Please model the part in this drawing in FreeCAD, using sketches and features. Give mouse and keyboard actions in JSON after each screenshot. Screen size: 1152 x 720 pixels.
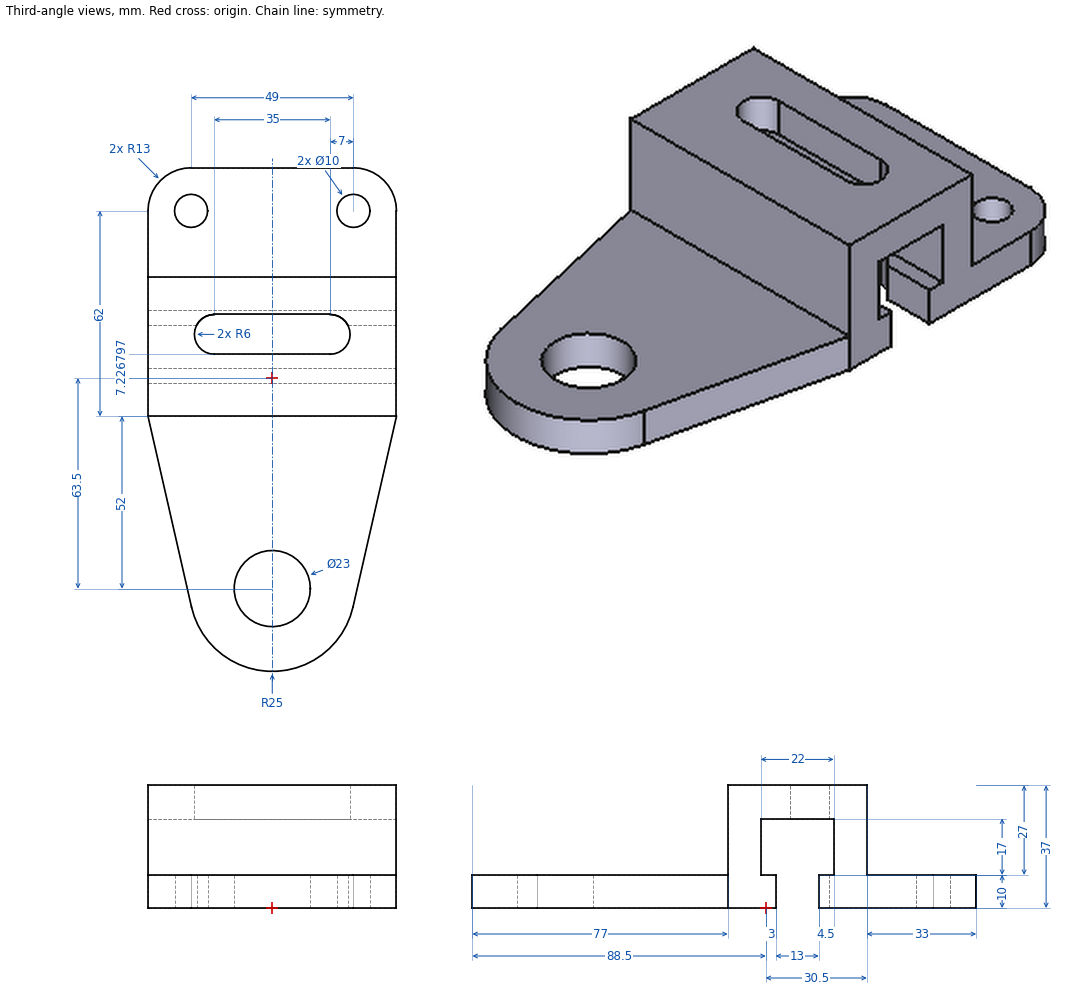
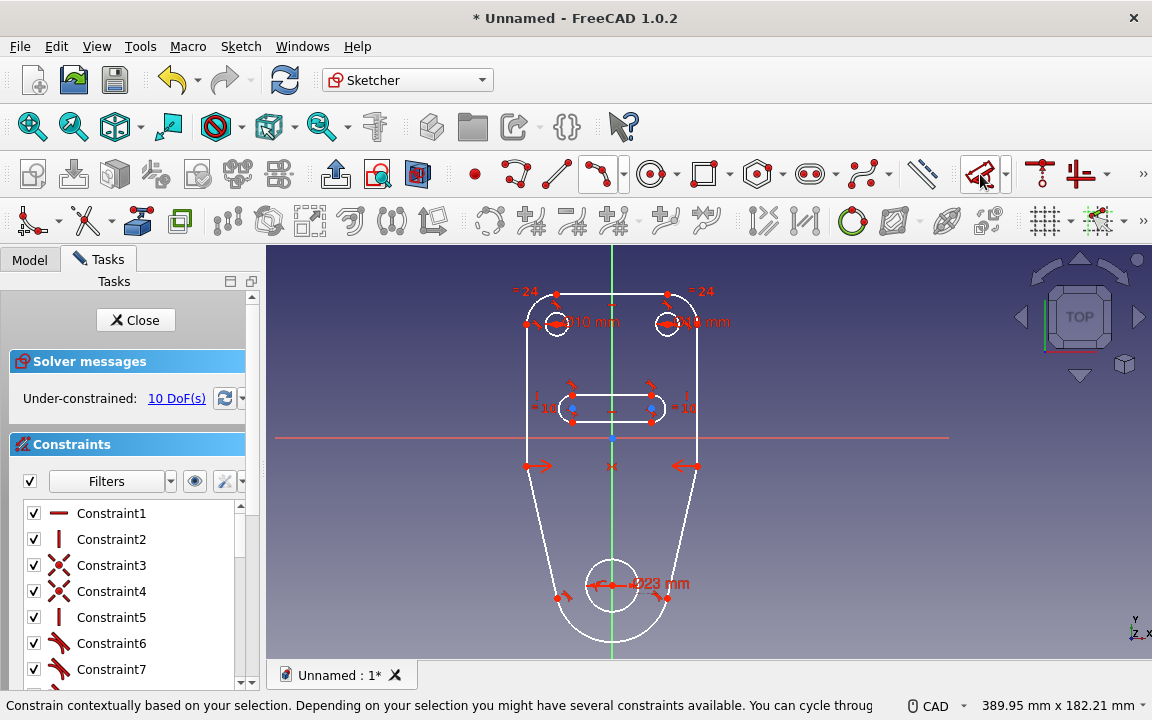
{"action": "scroll", "coordinate": [543, 298], "scroll_direction": "up", "scroll_amount": 2}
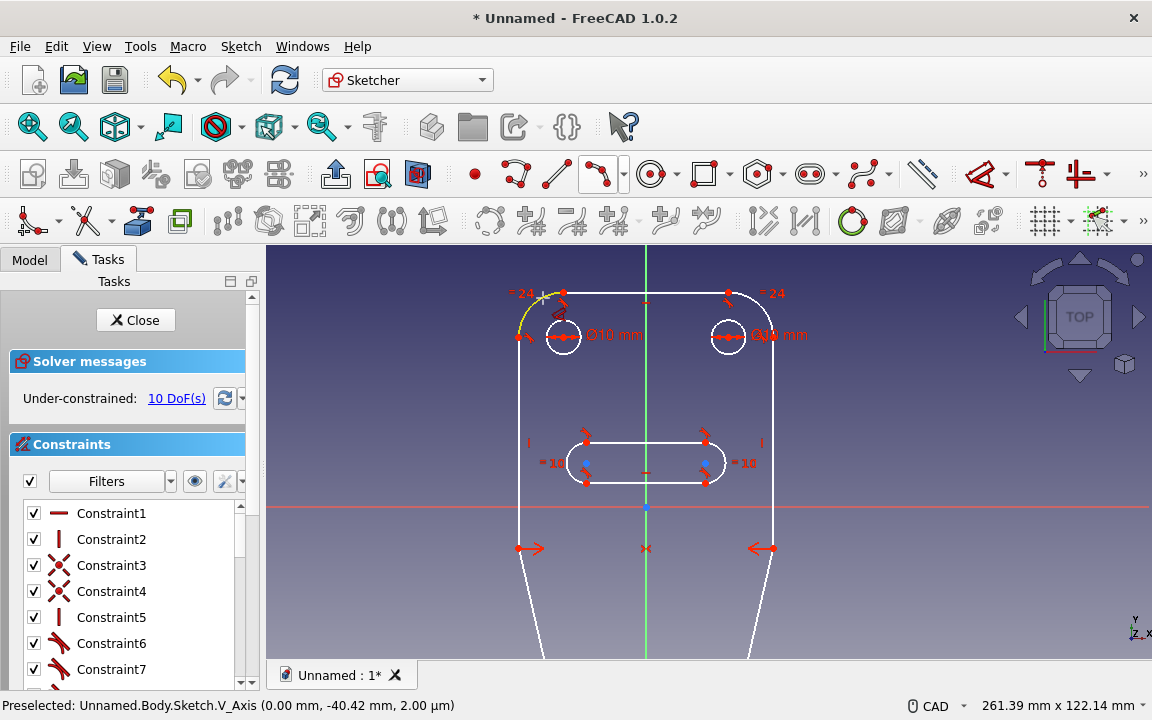
{"action": "left_click", "coordinate": [543, 297]}
{"action": "left_click", "coordinate": [500, 294]}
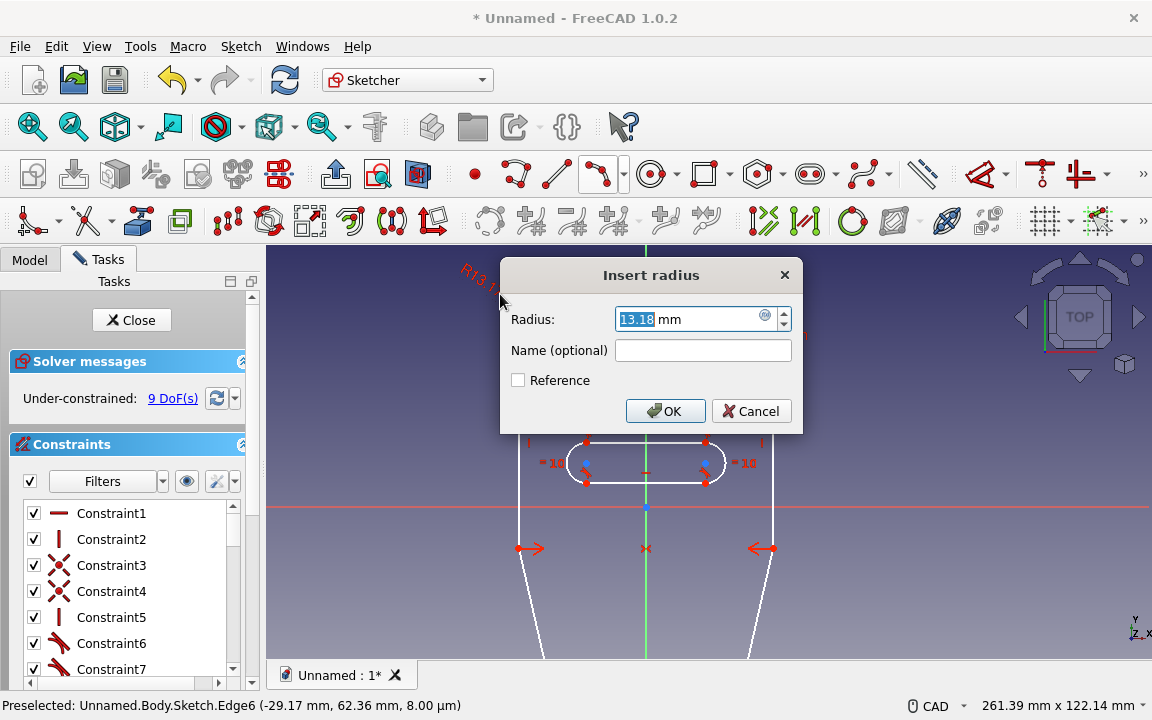
{"action": "type", "text": "13"}
{"action": "key", "text": "Return"}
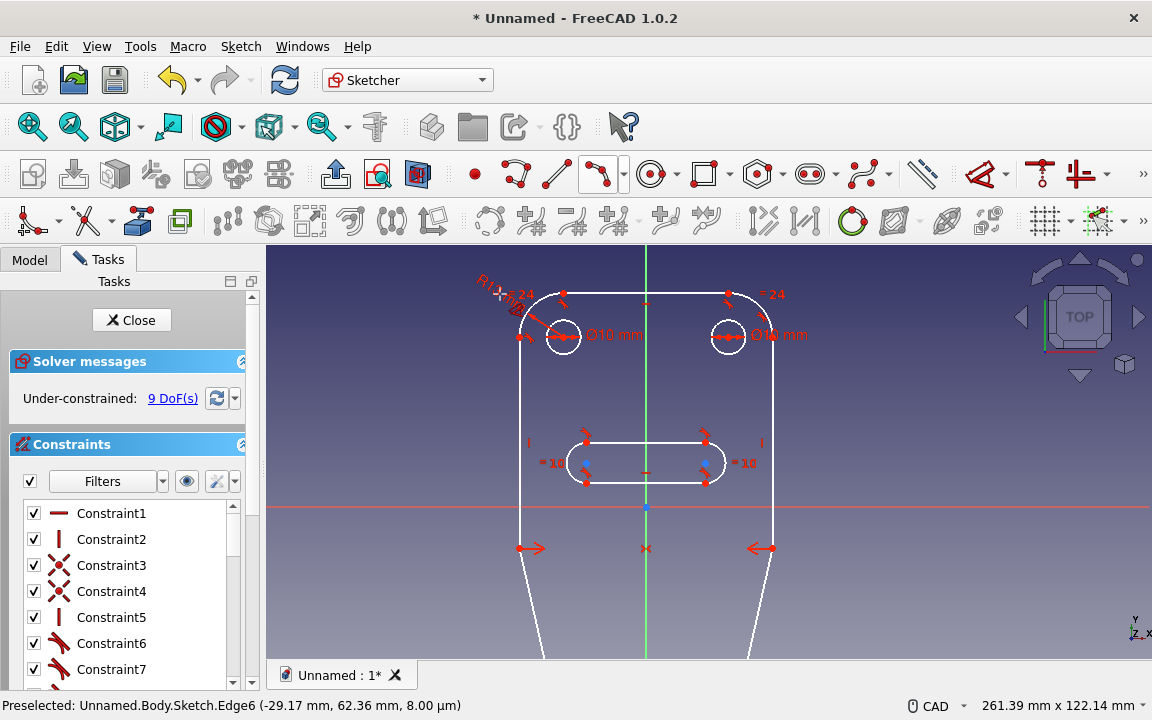
{"action": "scroll", "coordinate": [636, 373], "scroll_direction": "down", "scroll_amount": 4}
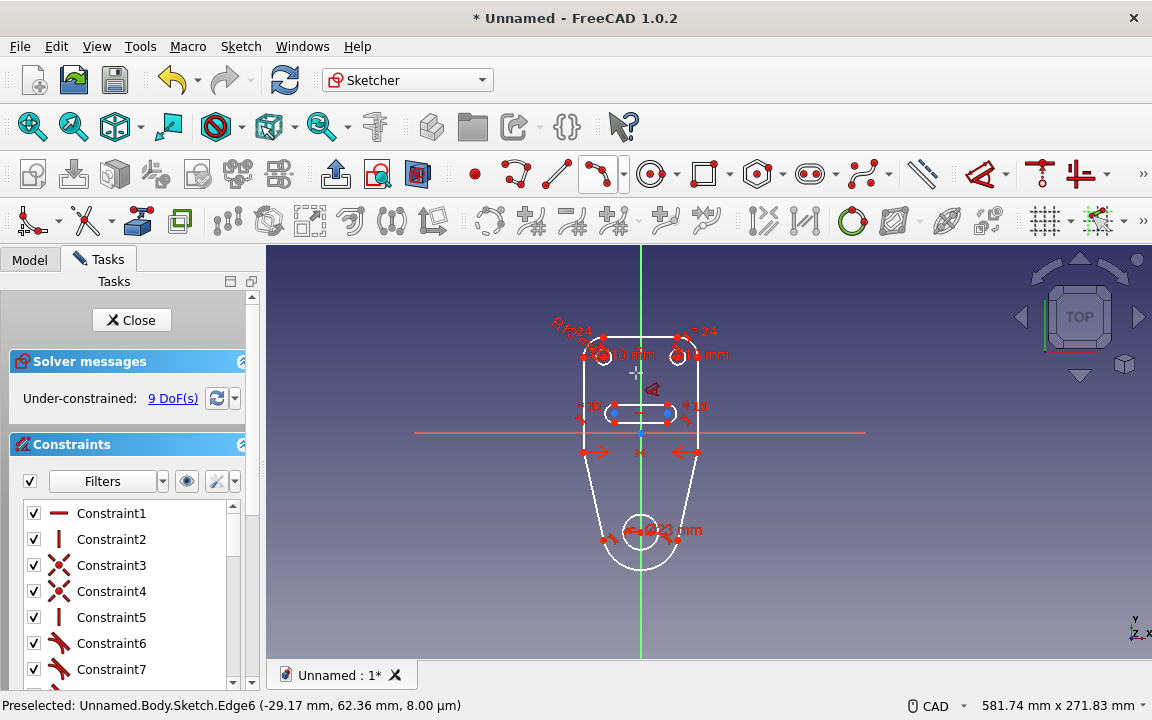
{"action": "left_click", "coordinate": [621, 565]}
{"action": "left_click", "coordinate": [604, 592]}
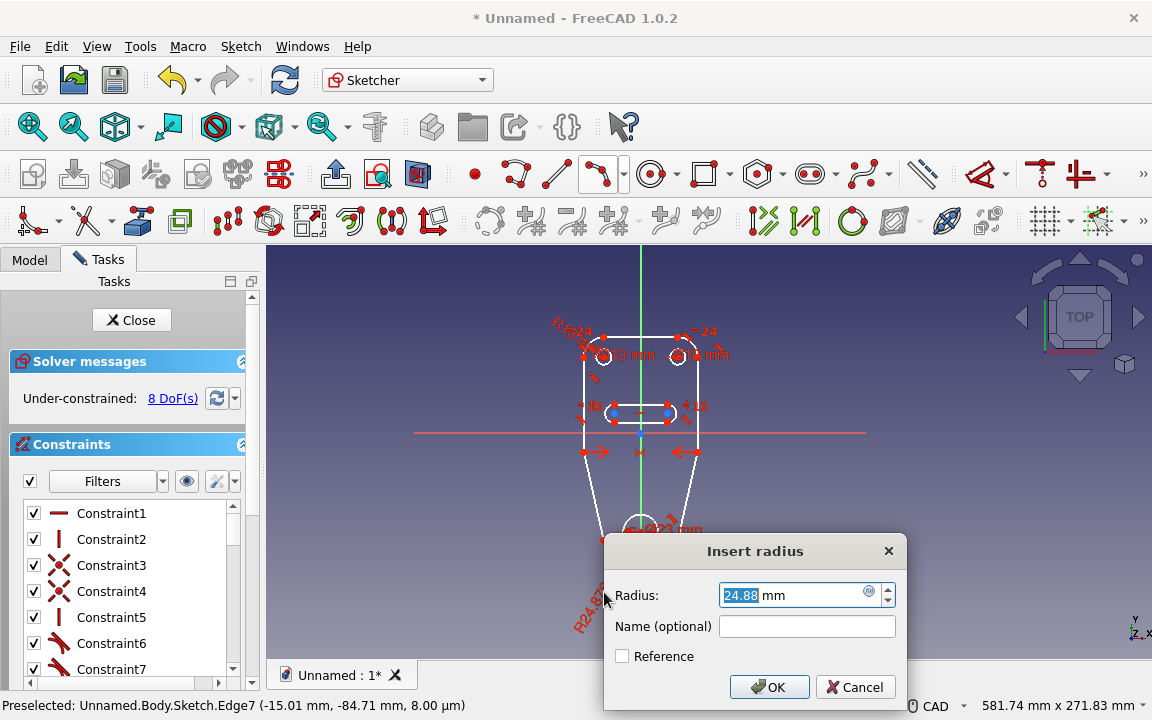
{"action": "type", "text": "25"}
{"action": "key", "text": "Return"}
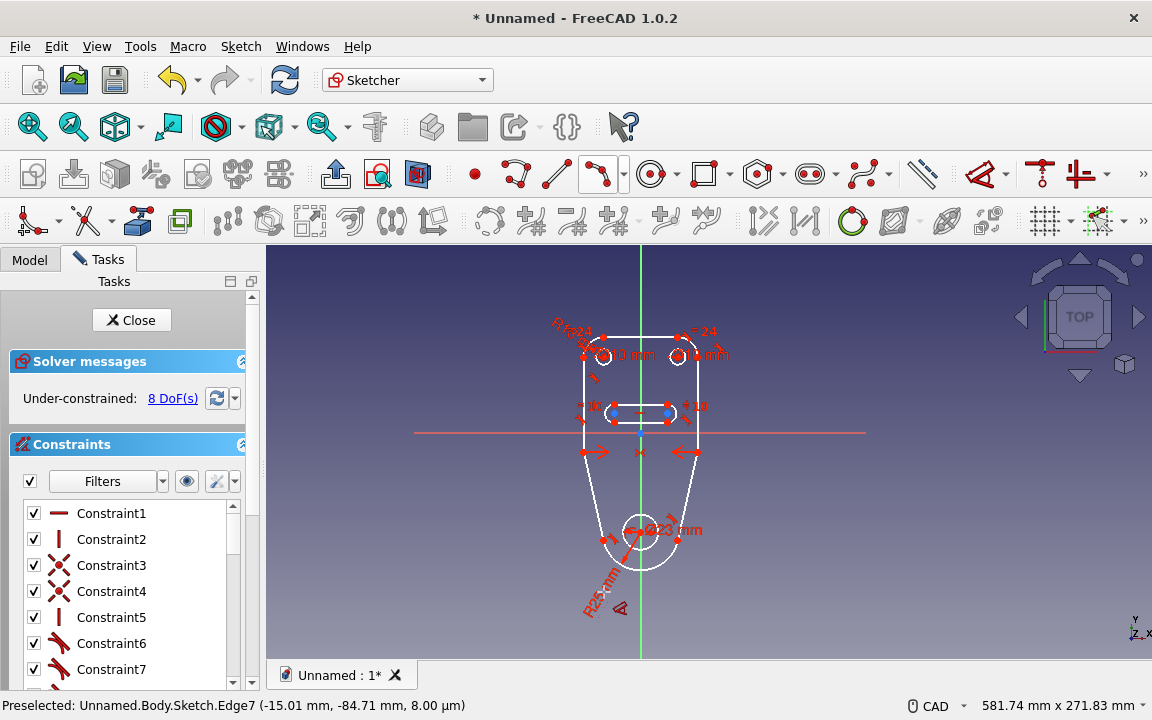
{"action": "scroll", "coordinate": [605, 414], "scroll_direction": "up", "scroll_amount": 8}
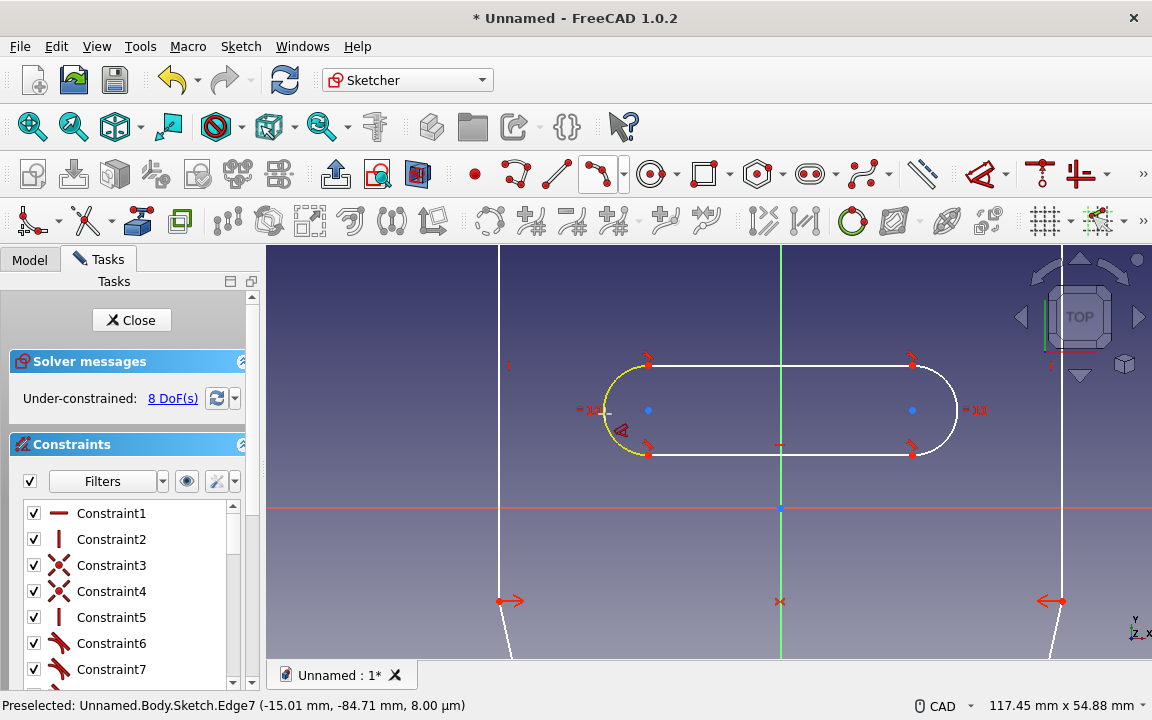
{"action": "left_click", "coordinate": [604, 411]}
{"action": "left_click", "coordinate": [572, 411]}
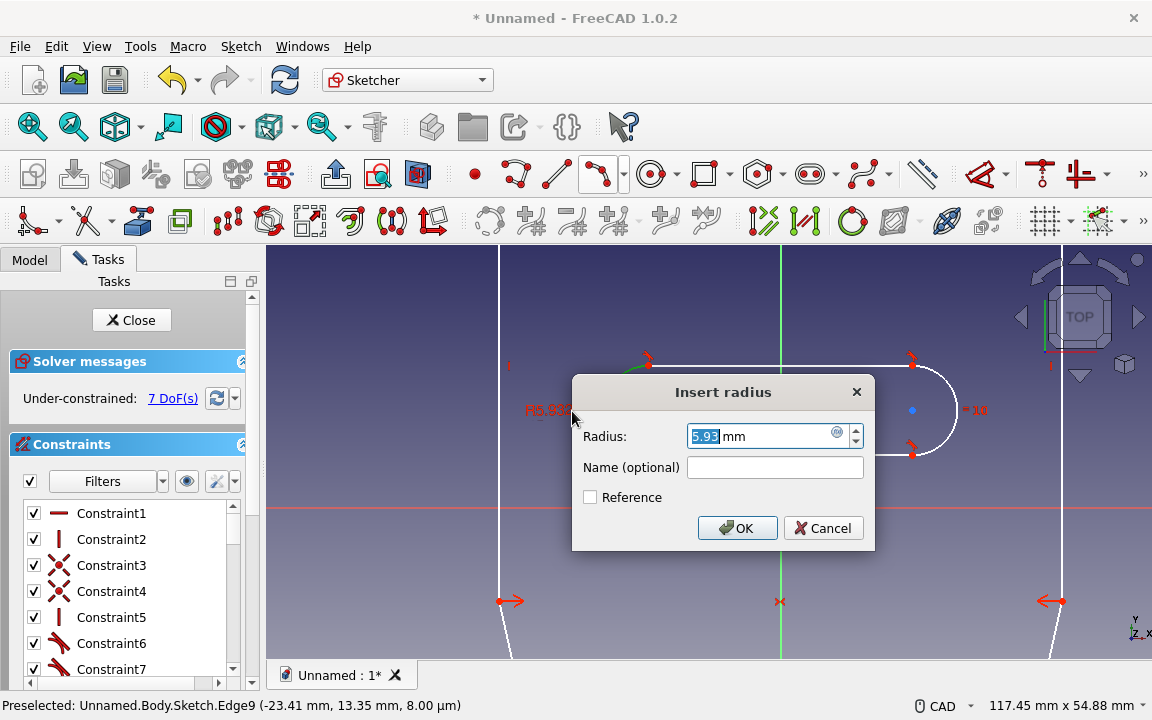
{"action": "type", "text": "6"}
{"action": "key", "text": "Return"}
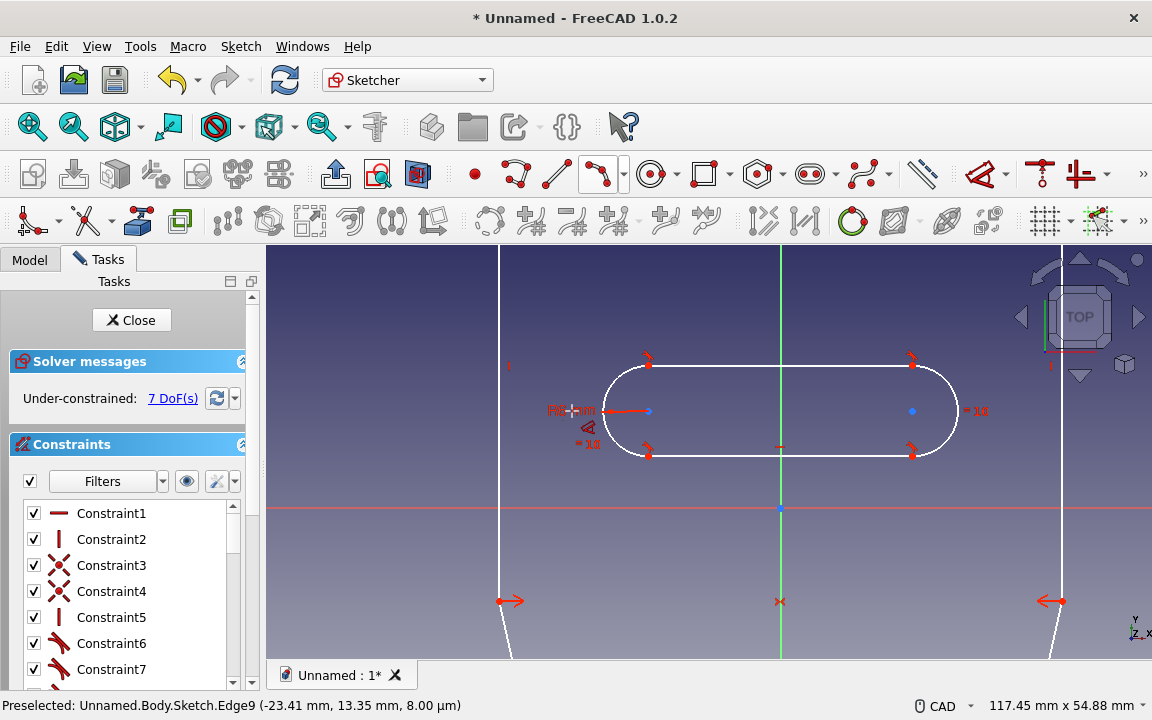
{"action": "scroll", "coordinate": [605, 414], "scroll_direction": "down", "scroll_amount": 8}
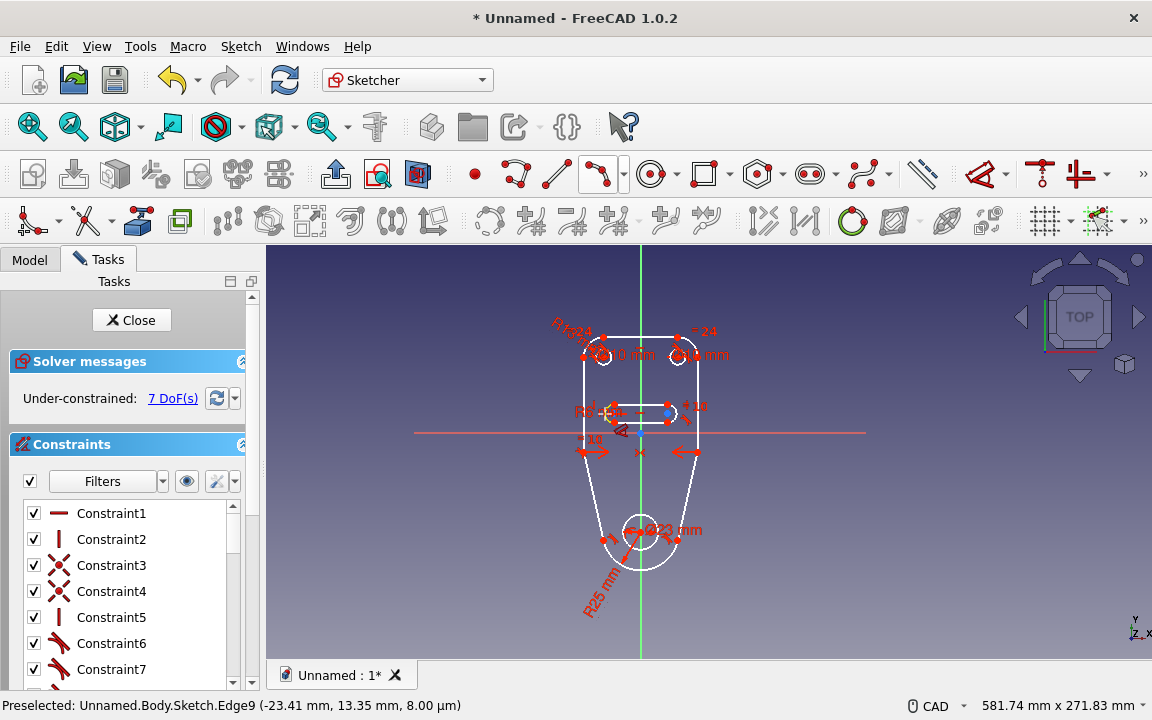
{"action": "left_click", "coordinate": [656, 337]}
{"action": "left_click", "coordinate": [624, 303]}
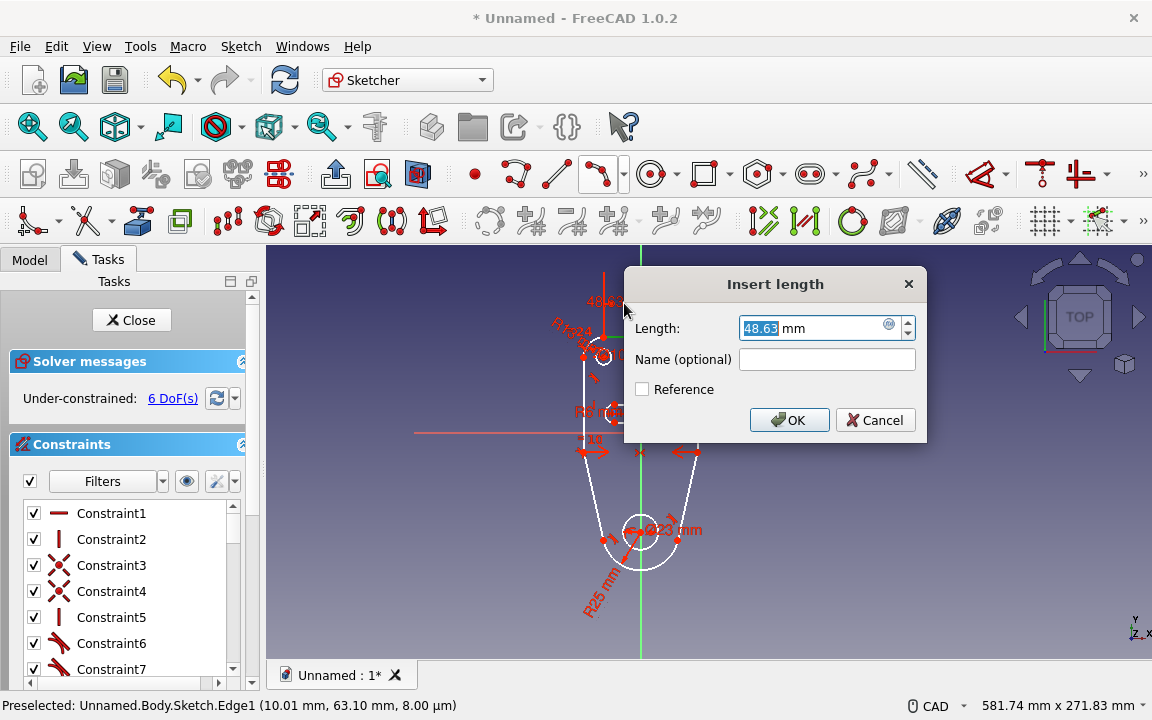
{"action": "type", "text": "49"}
{"action": "key", "text": "Return"}